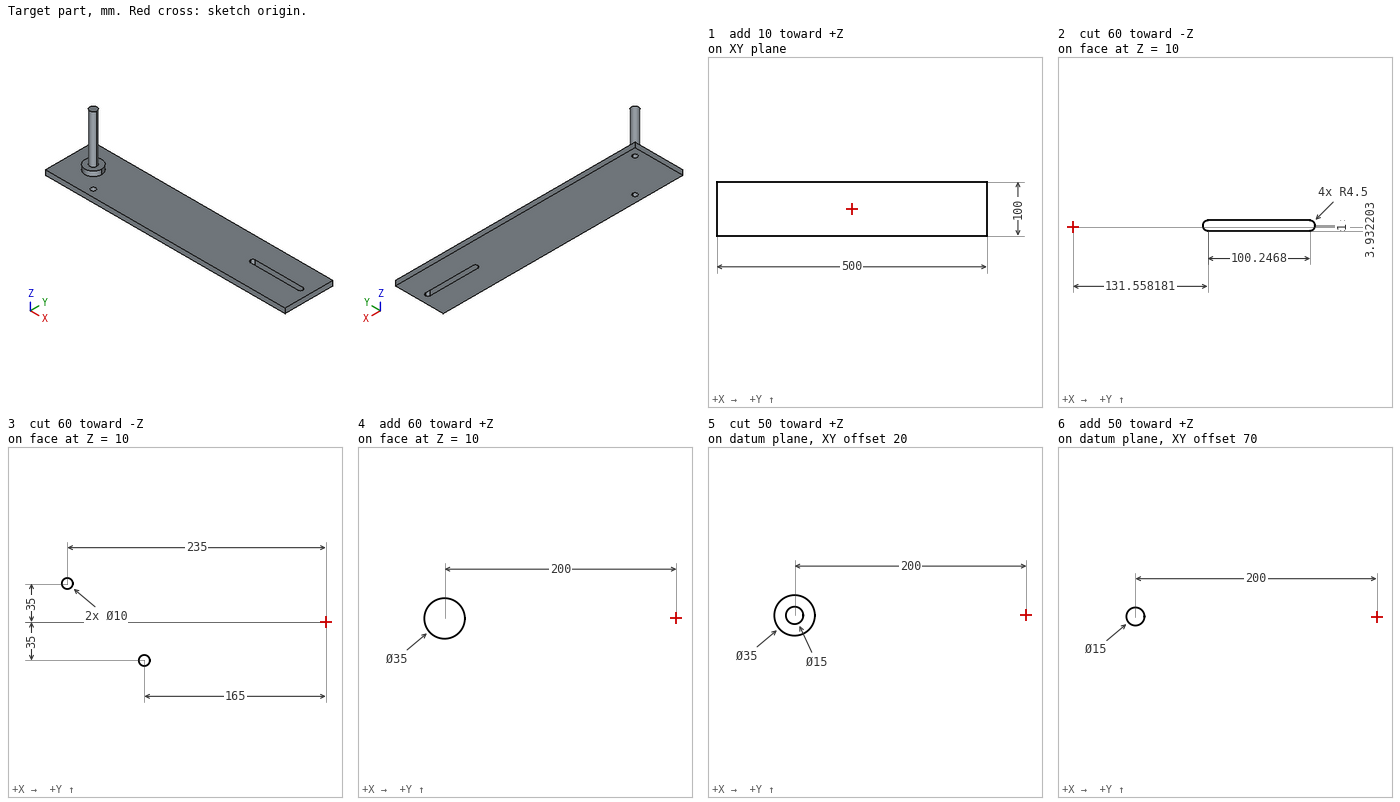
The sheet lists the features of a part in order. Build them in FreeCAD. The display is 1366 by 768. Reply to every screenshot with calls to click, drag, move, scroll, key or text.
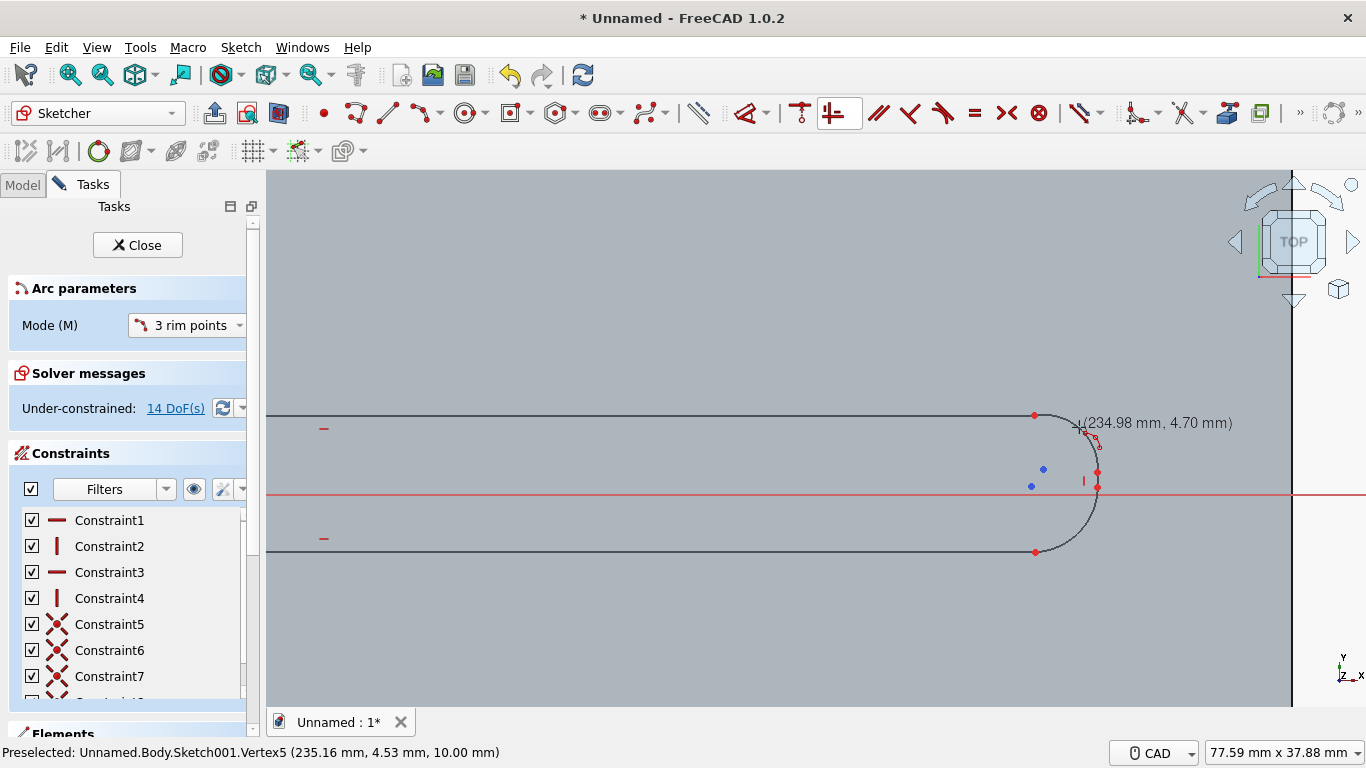
scroll(1083, 428, down, 8)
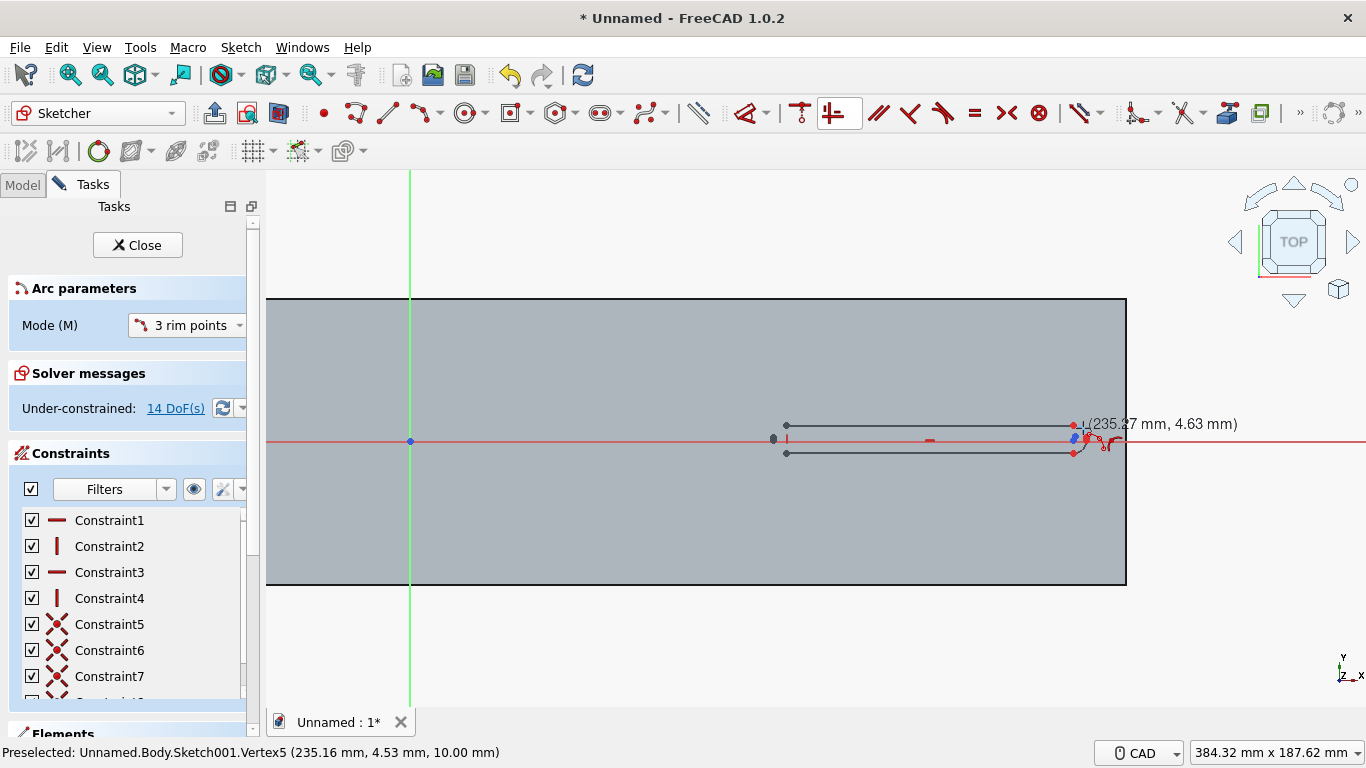
click(787, 426)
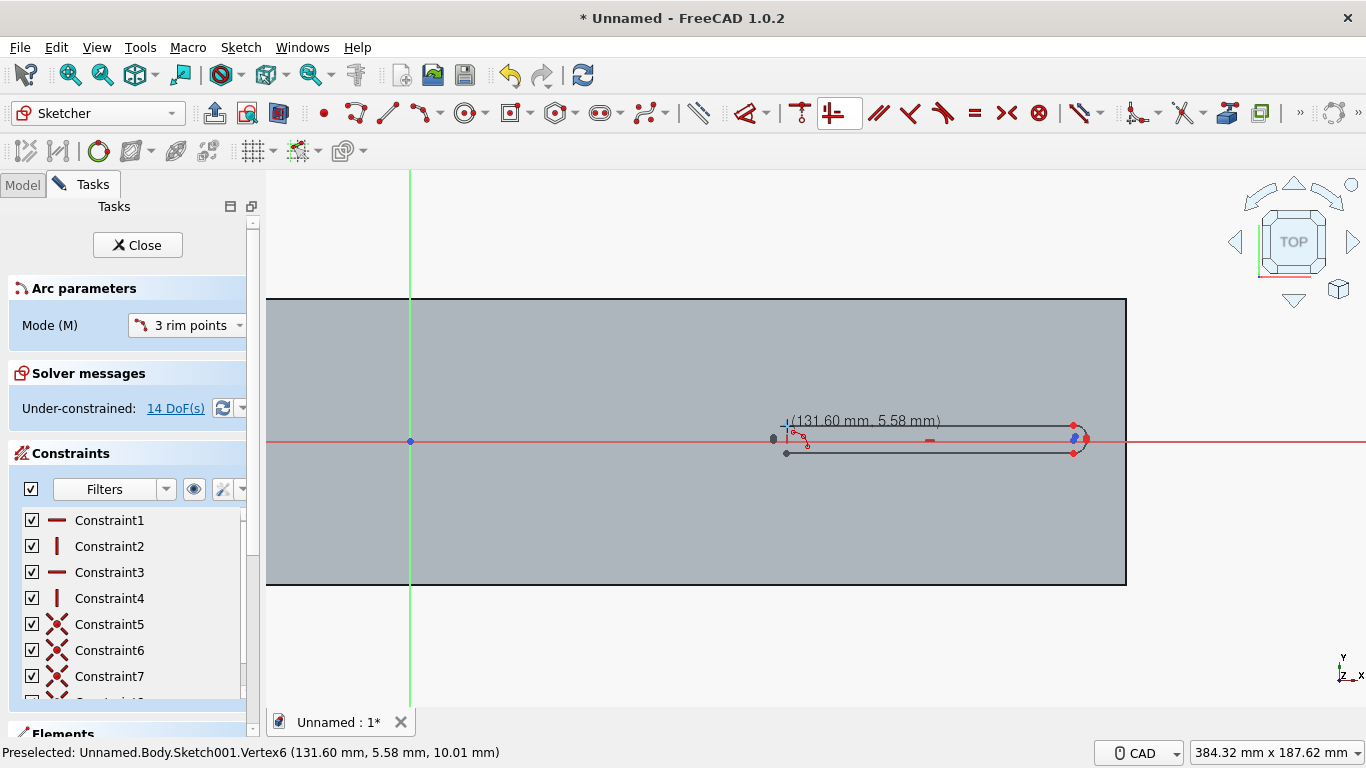
scroll(774, 437, up, 13)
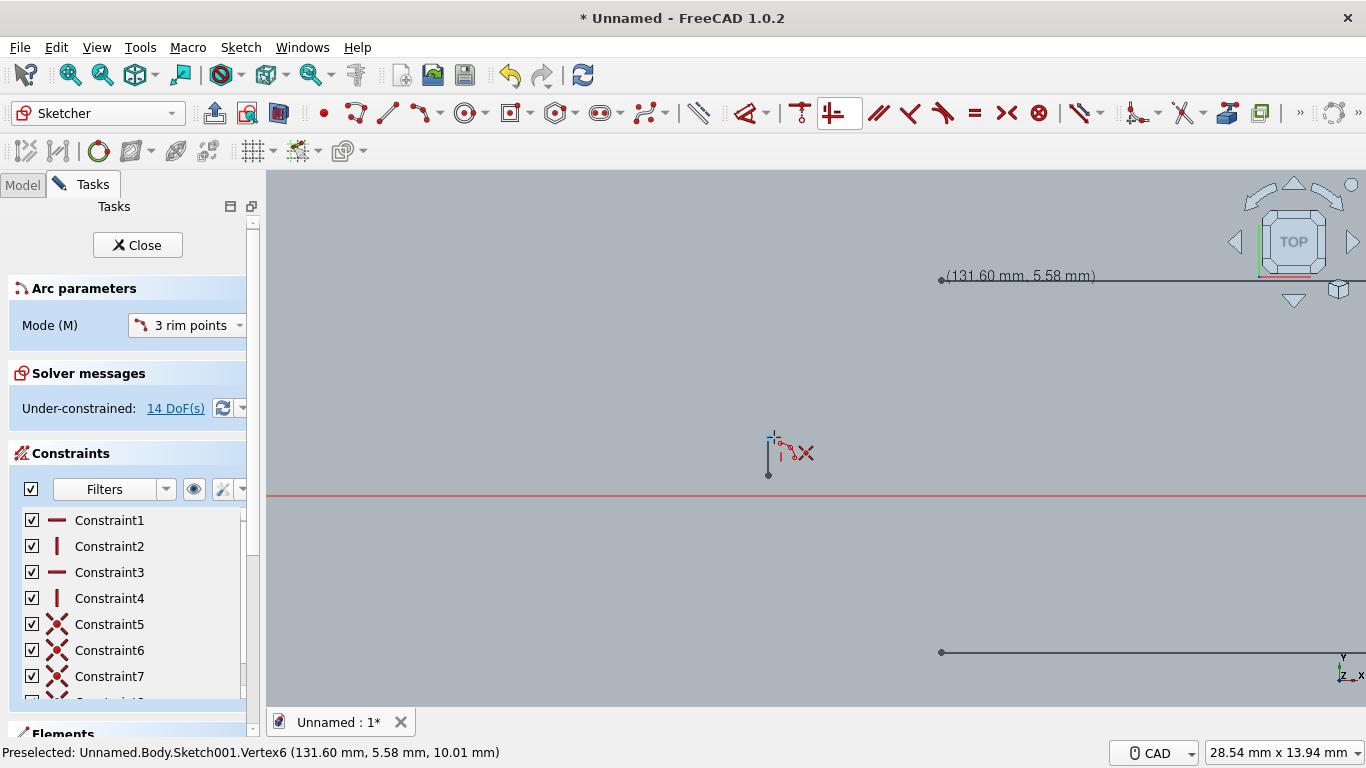
click(768, 437)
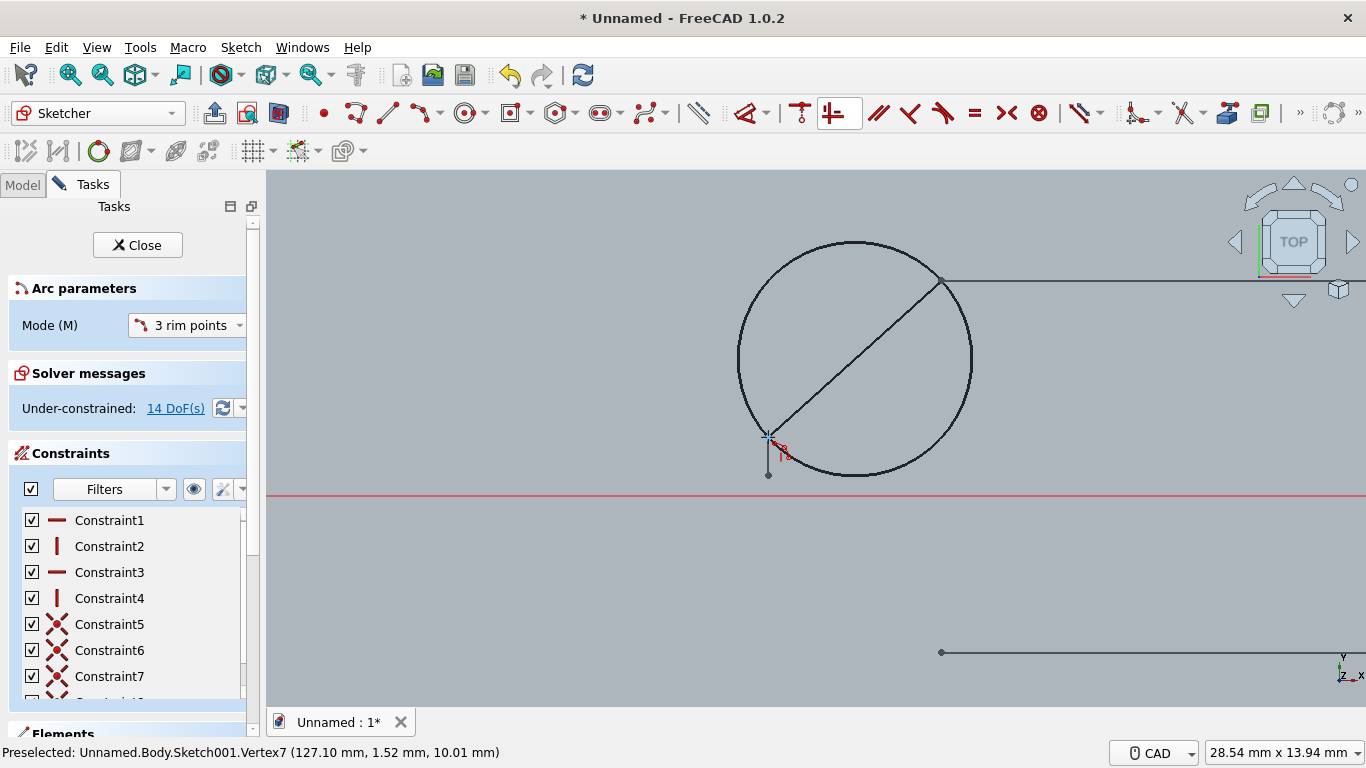
scroll(773, 437, down, 13)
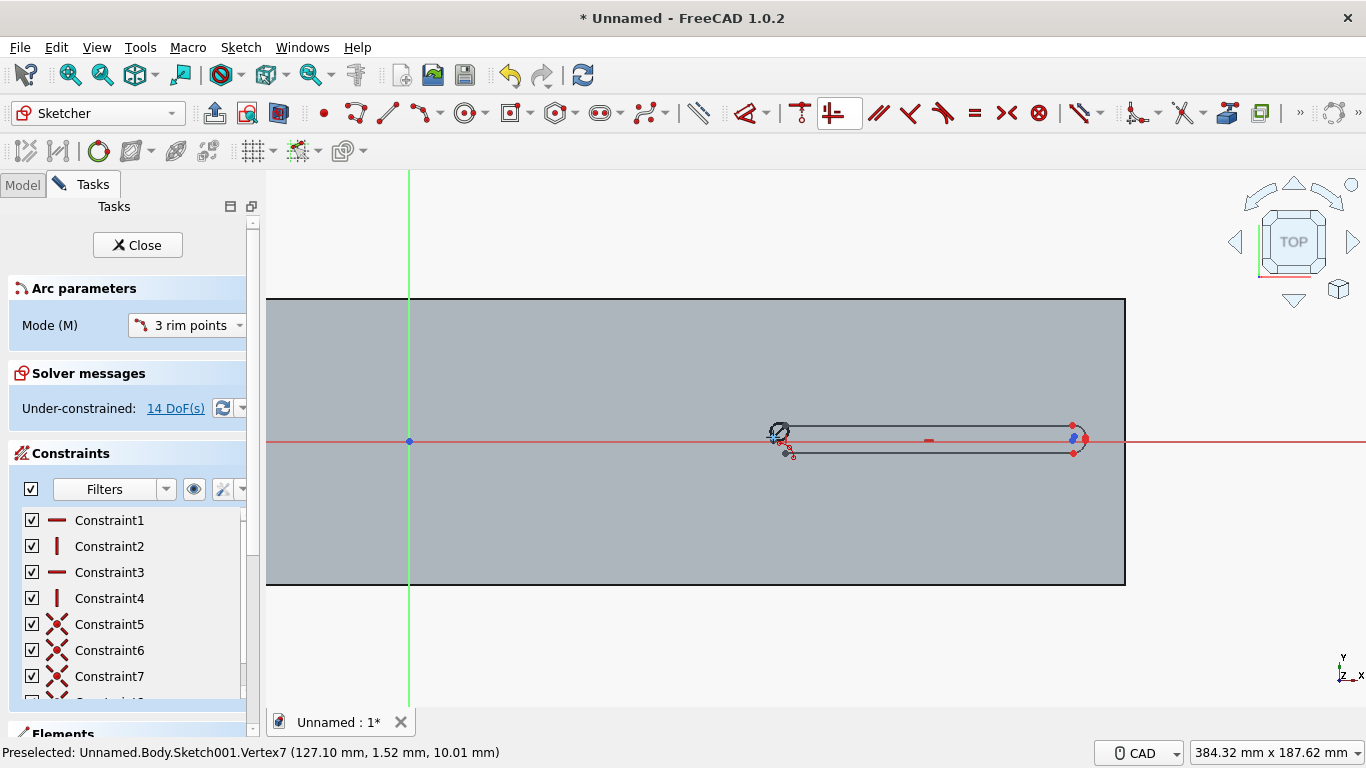
scroll(777, 428, up, 8)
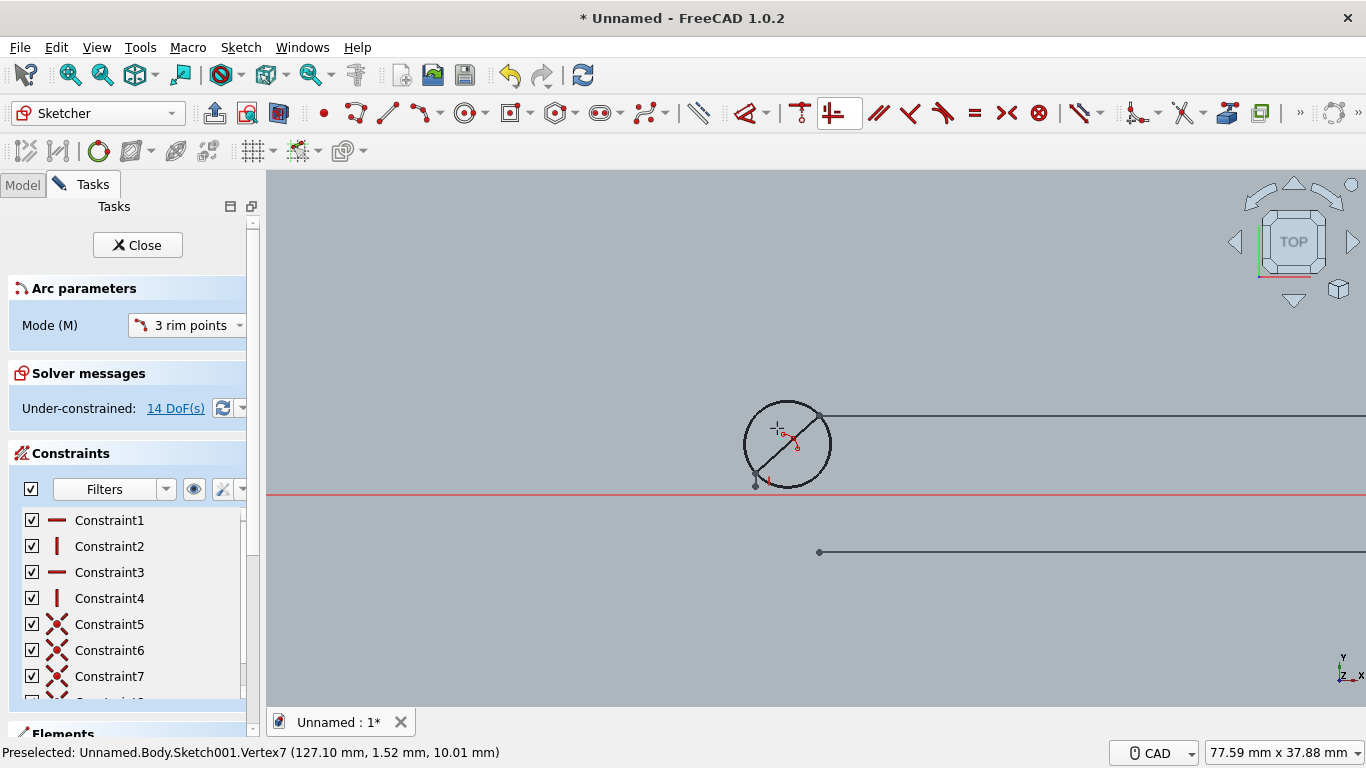
click(774, 427)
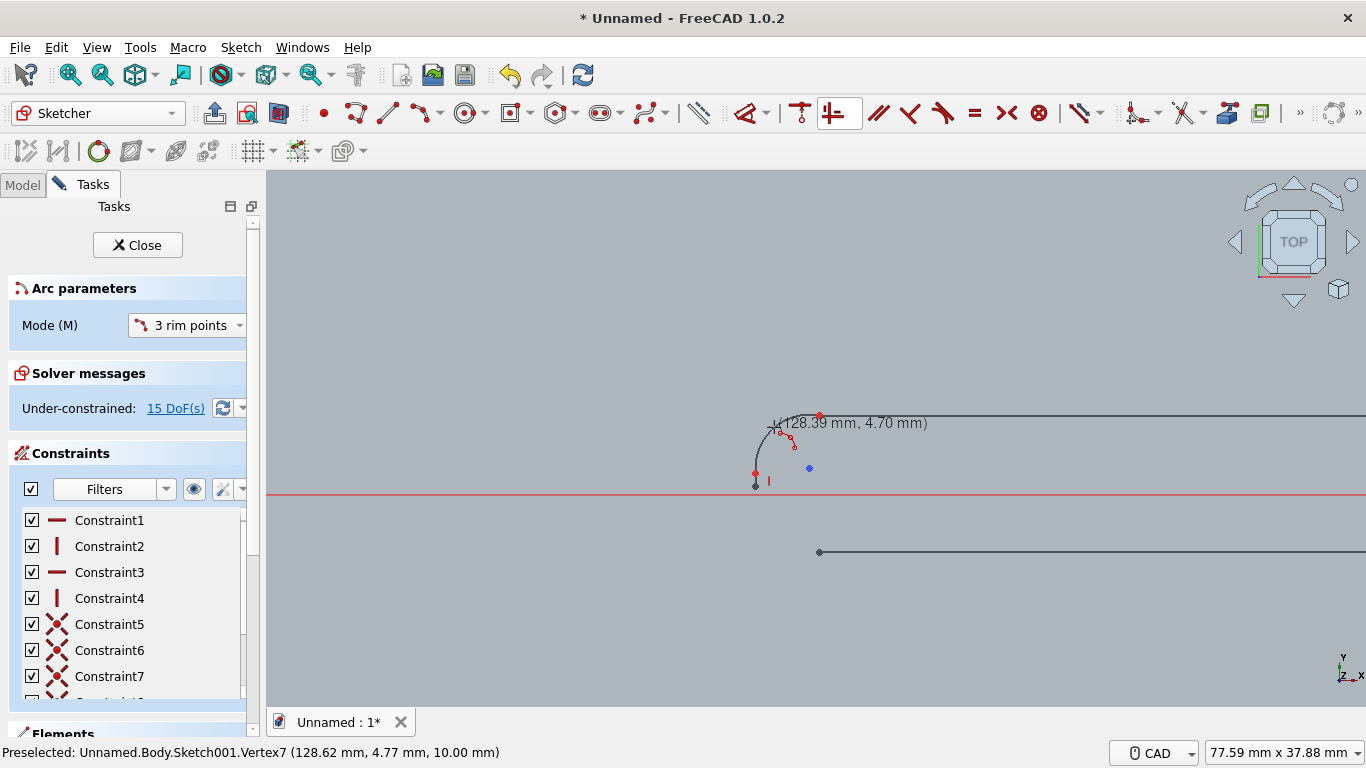
scroll(755, 487, up, 5)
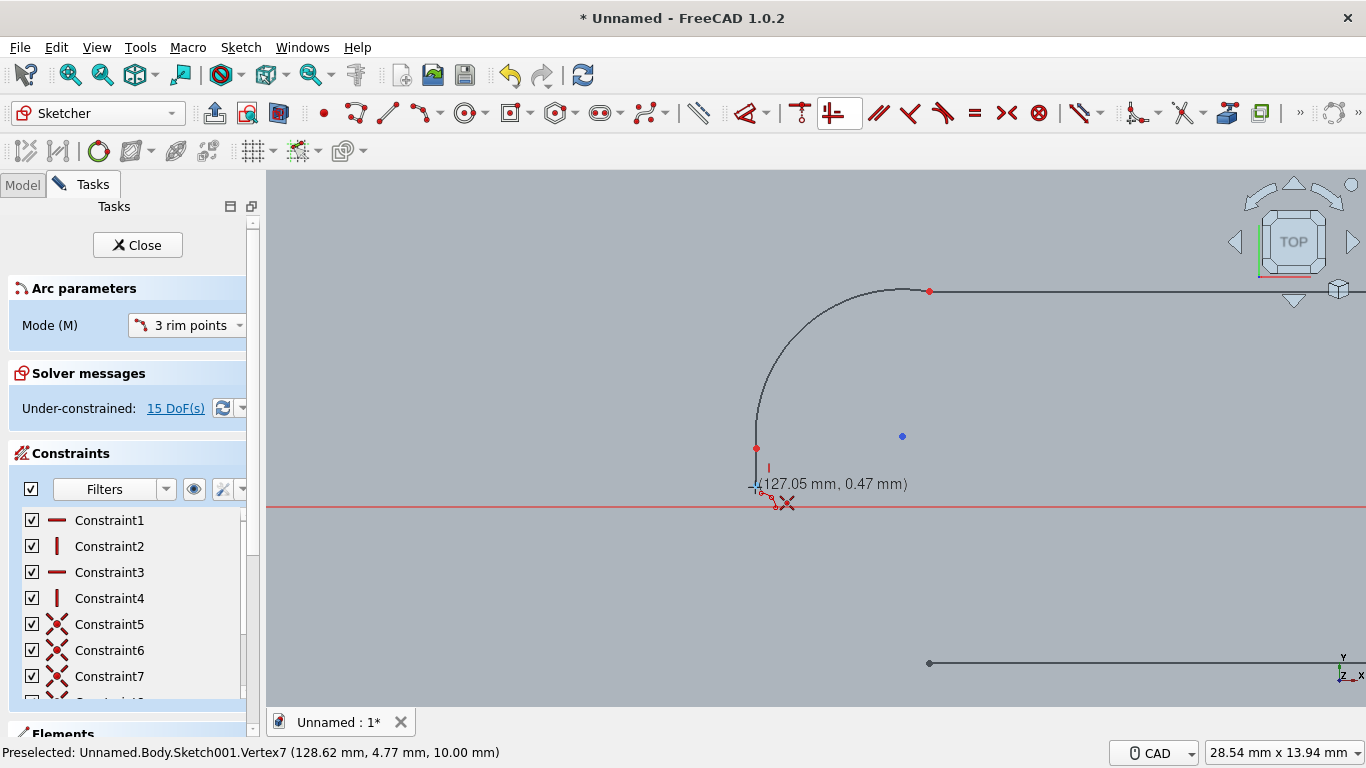
click(756, 486)